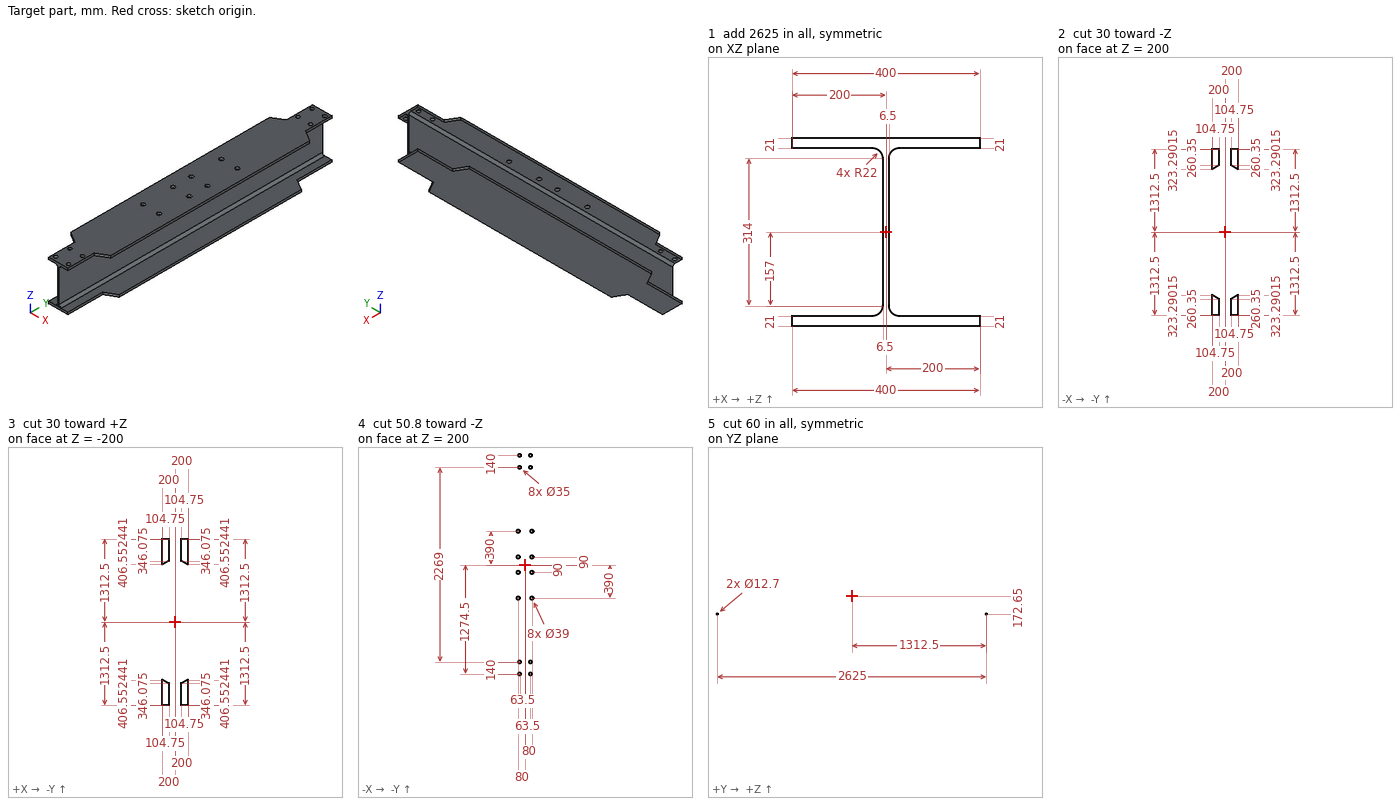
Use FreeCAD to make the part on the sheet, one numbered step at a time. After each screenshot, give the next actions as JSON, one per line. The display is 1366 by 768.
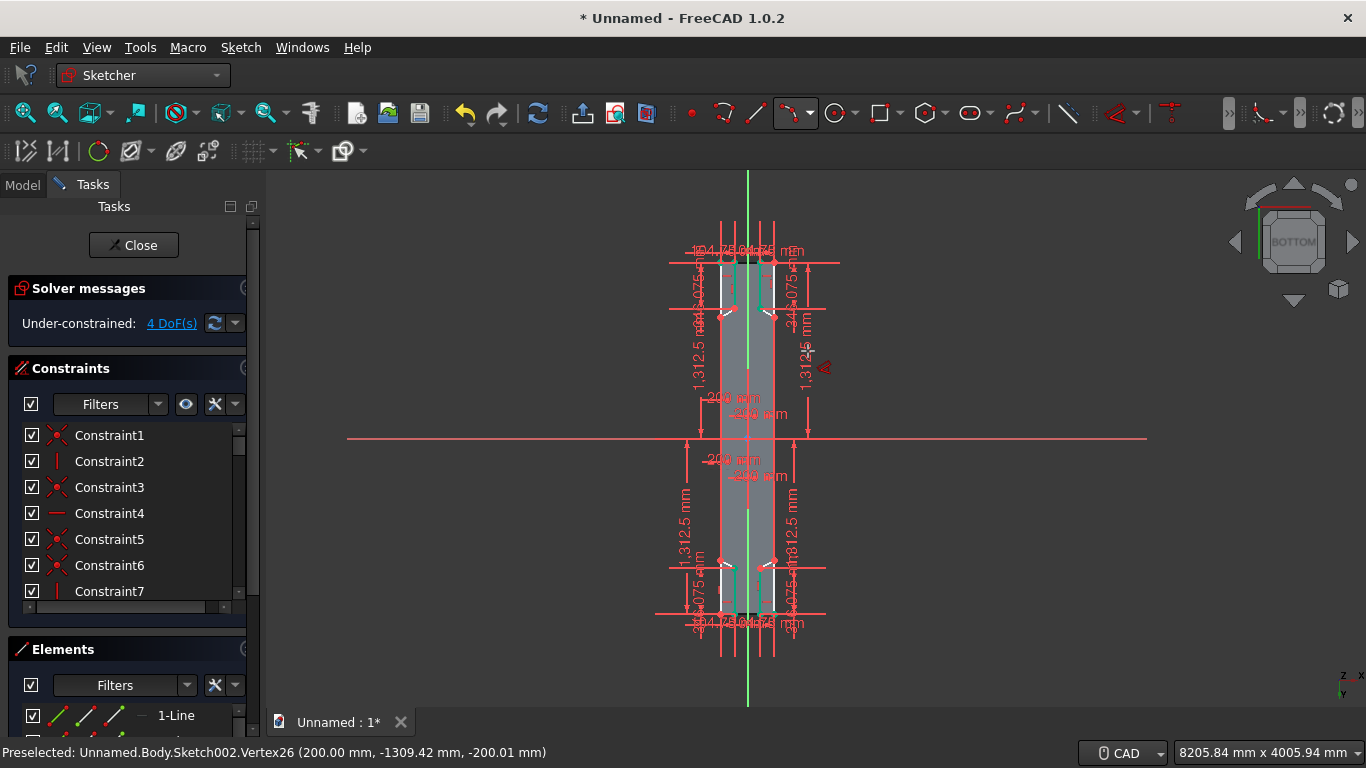
{"action": "left_click", "coordinate": [774, 598]}
{"action": "left_click", "coordinate": [808, 569]}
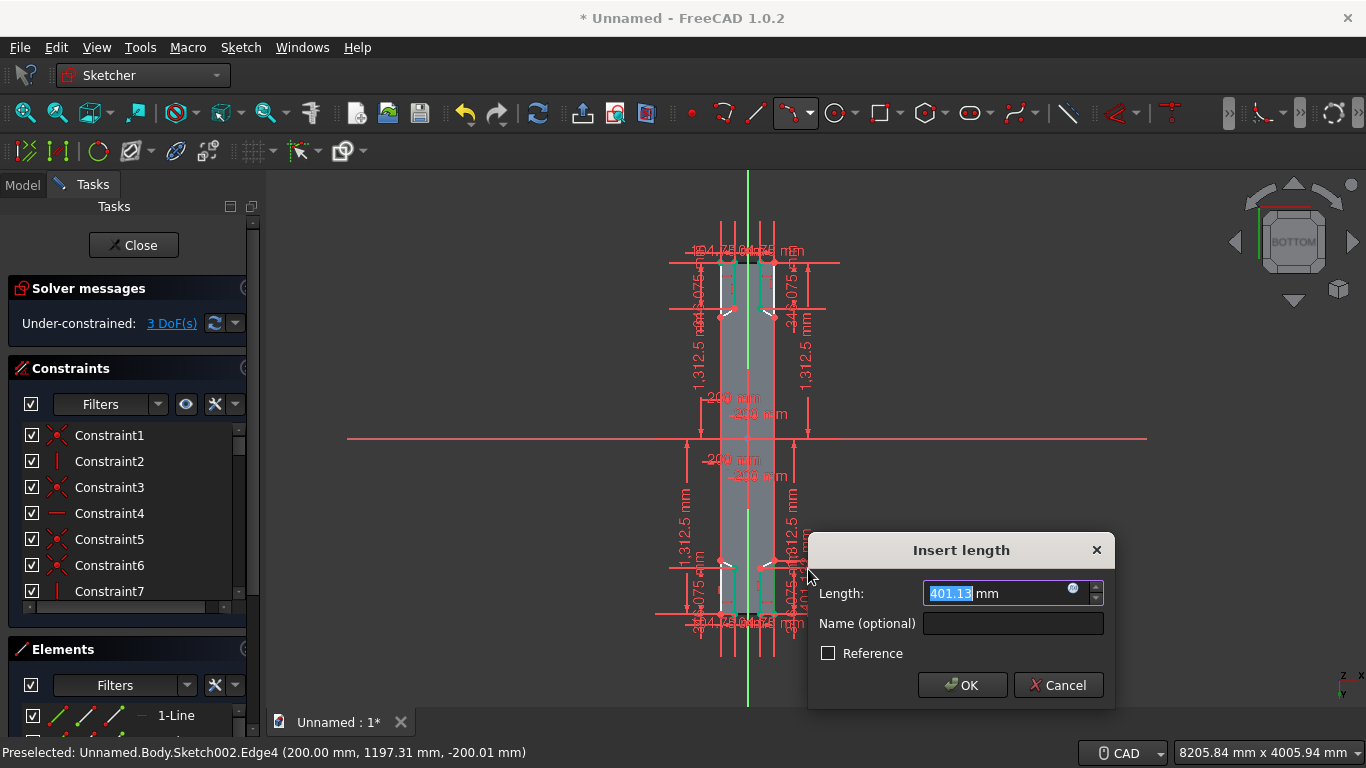
{"action": "type", "text": "406.552441"}
{"action": "key", "text": "Return"}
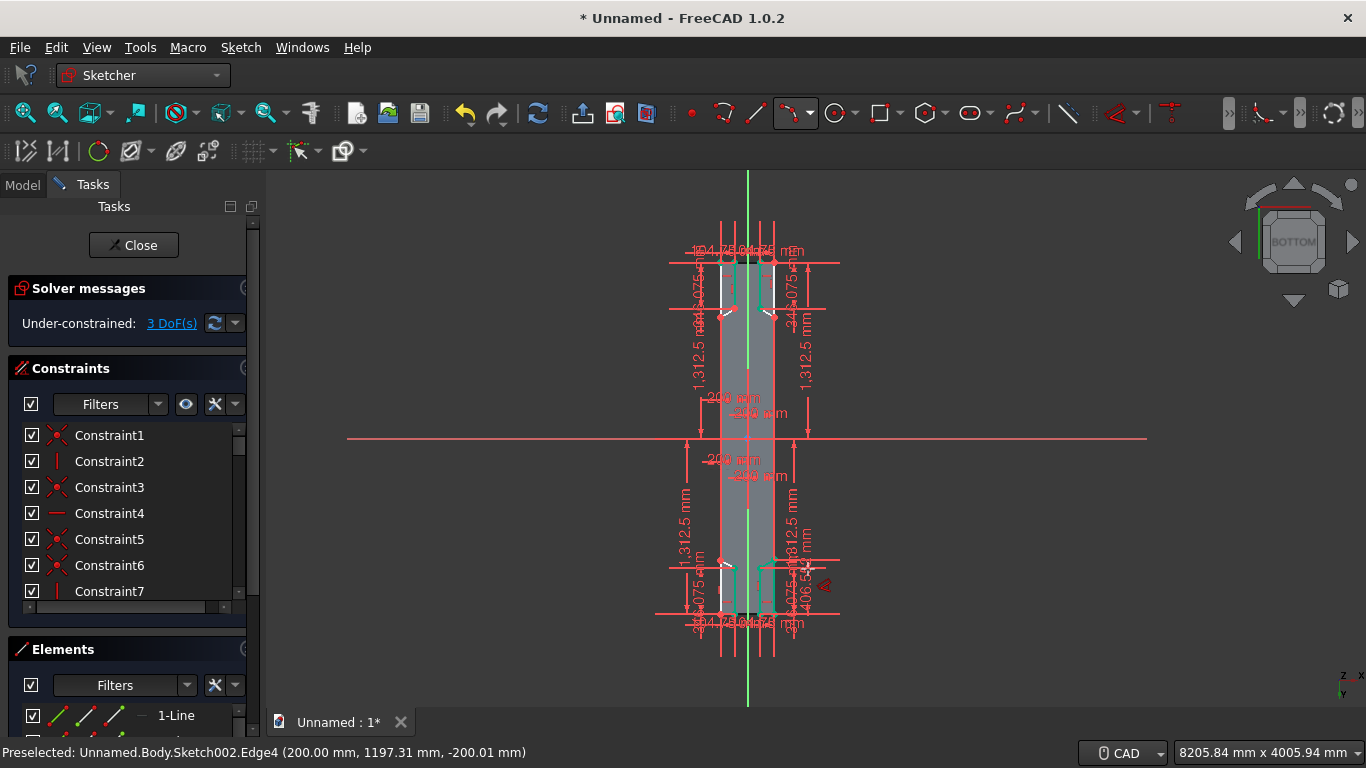
{"action": "left_click", "coordinate": [721, 577]}
{"action": "left_click", "coordinate": [687, 569]}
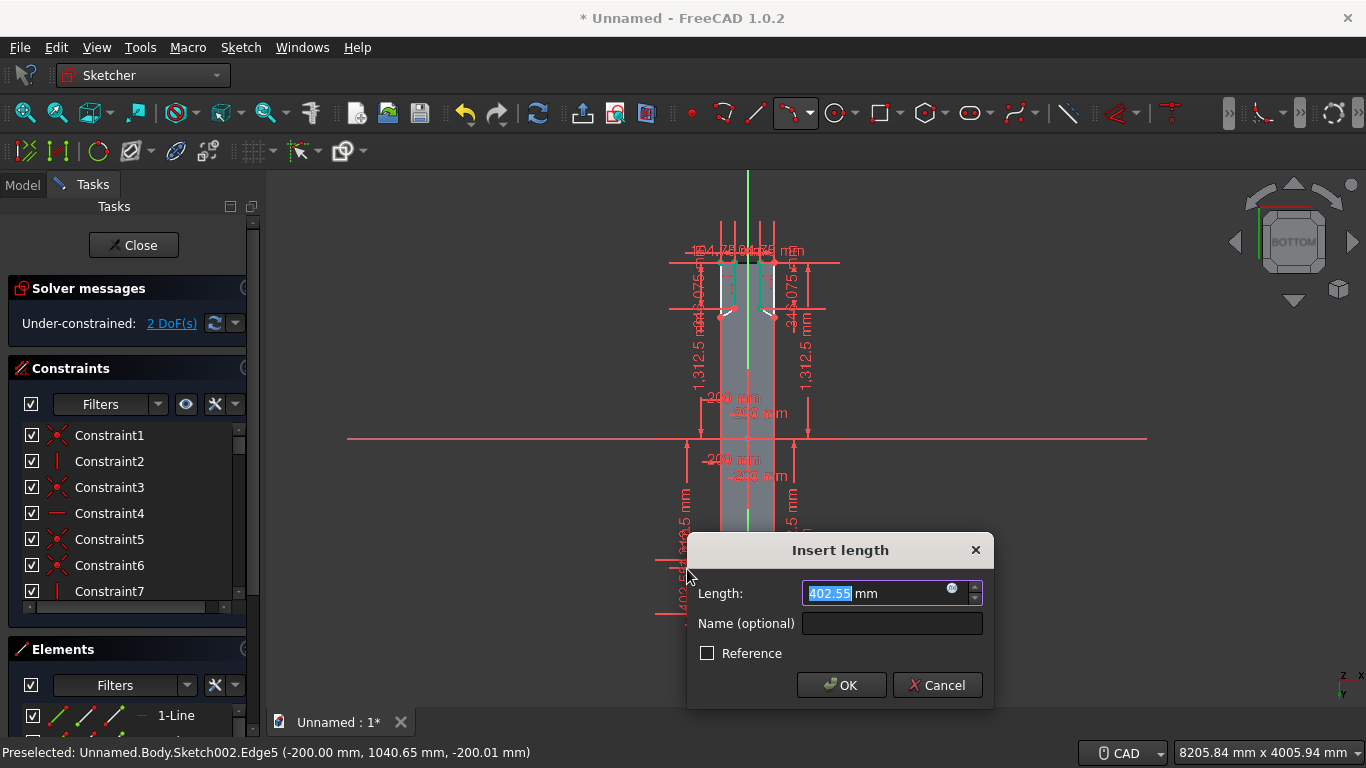
{"action": "type", "text": "406.552441"}
{"action": "key", "text": "Return"}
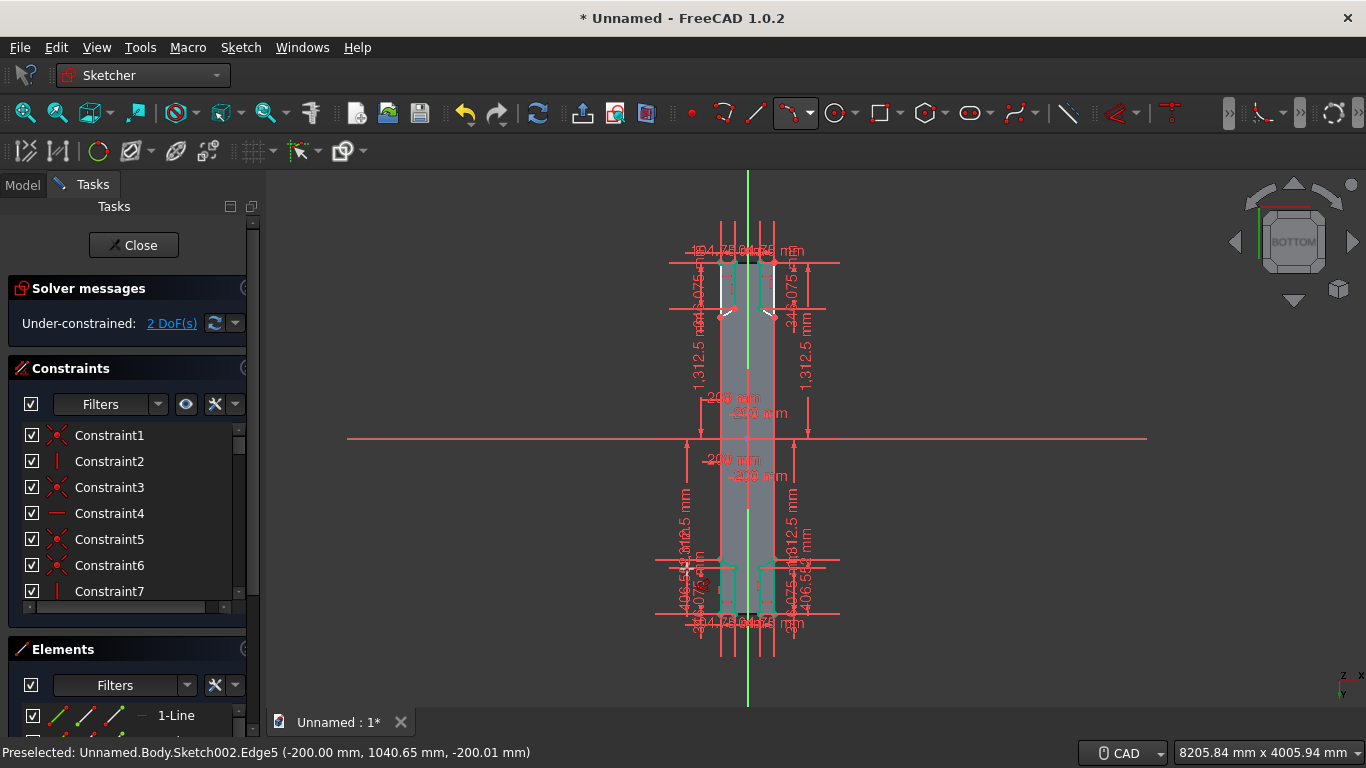
{"action": "left_click", "coordinate": [721, 279]}
{"action": "left_click", "coordinate": [687, 309]}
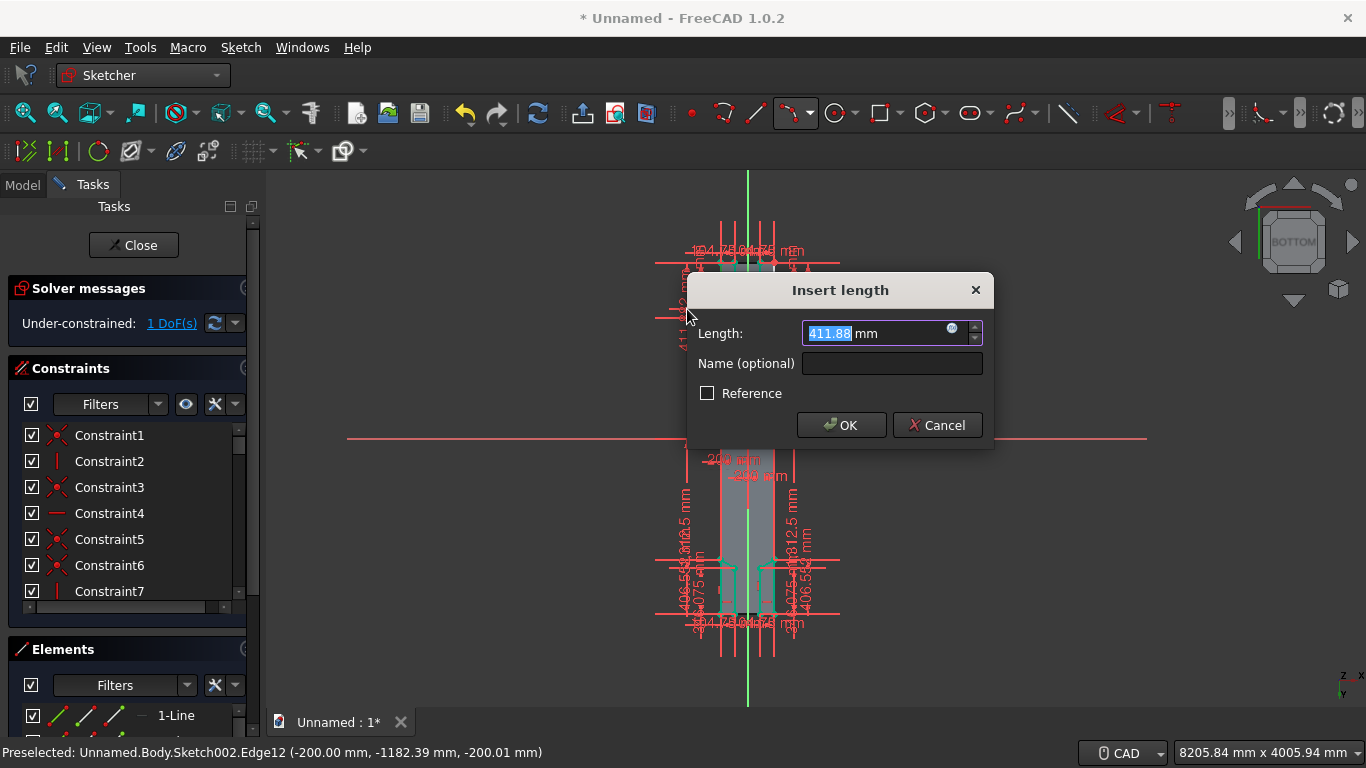
{"action": "type", "text": "406.552441"}
{"action": "key", "text": "Return"}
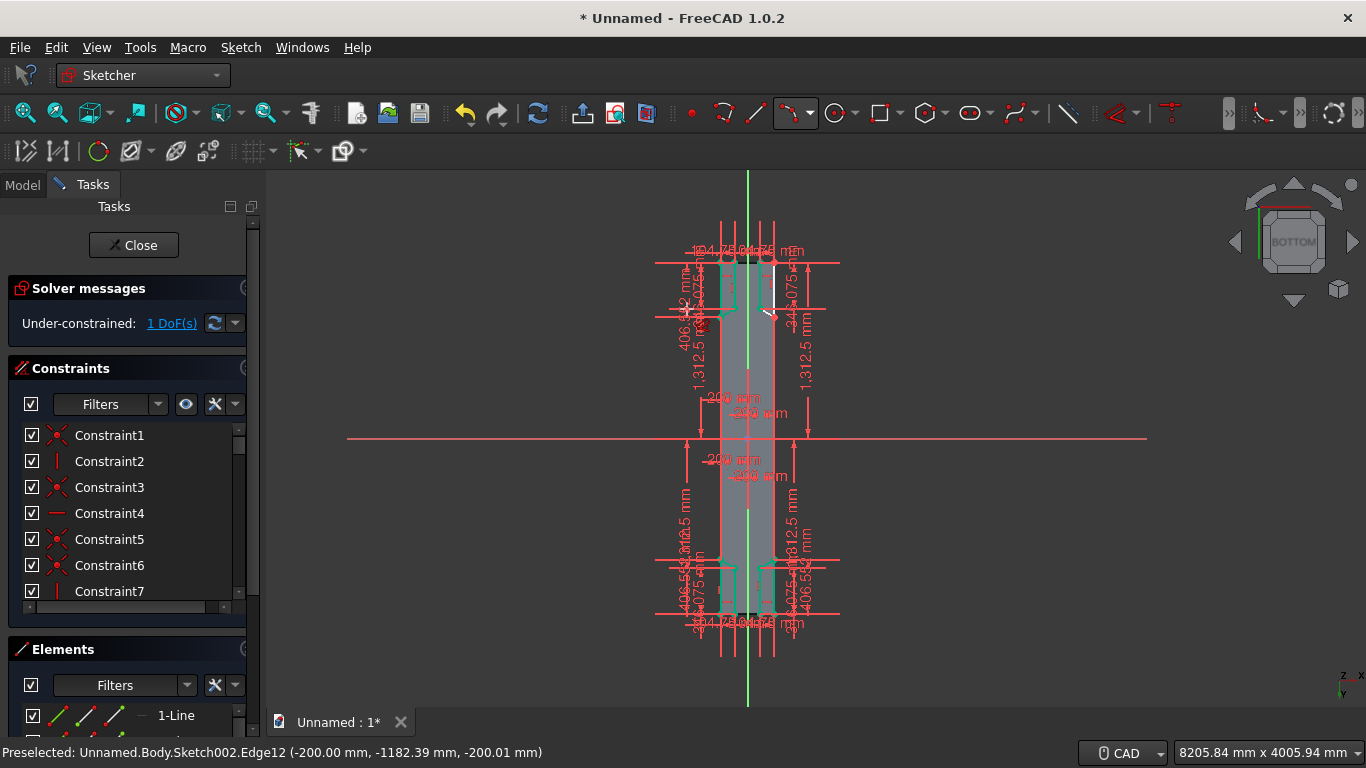
{"action": "left_click", "coordinate": [774, 301]}
{"action": "left_click", "coordinate": [808, 309]}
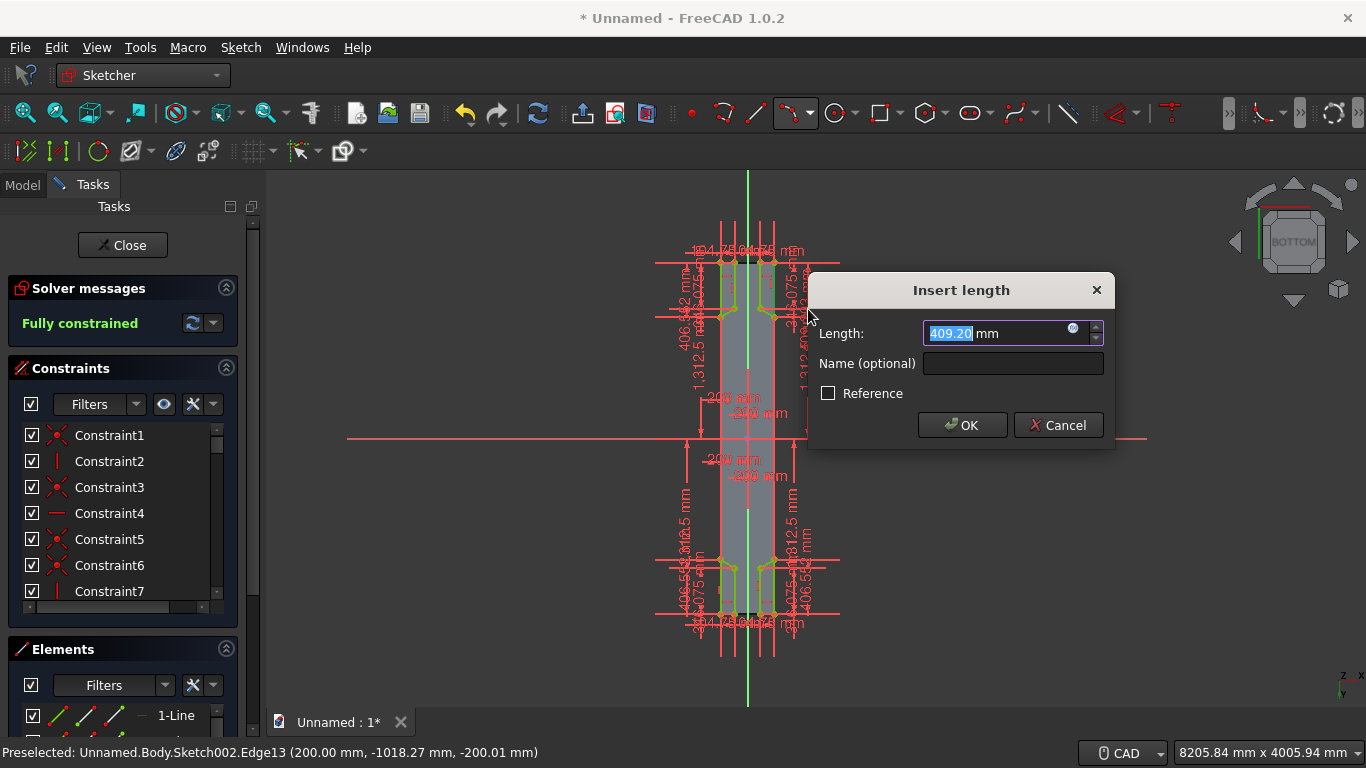
{"action": "type", "text": "406.552441"}
{"action": "key", "text": "Return"}
{"action": "key", "text": "Escape"}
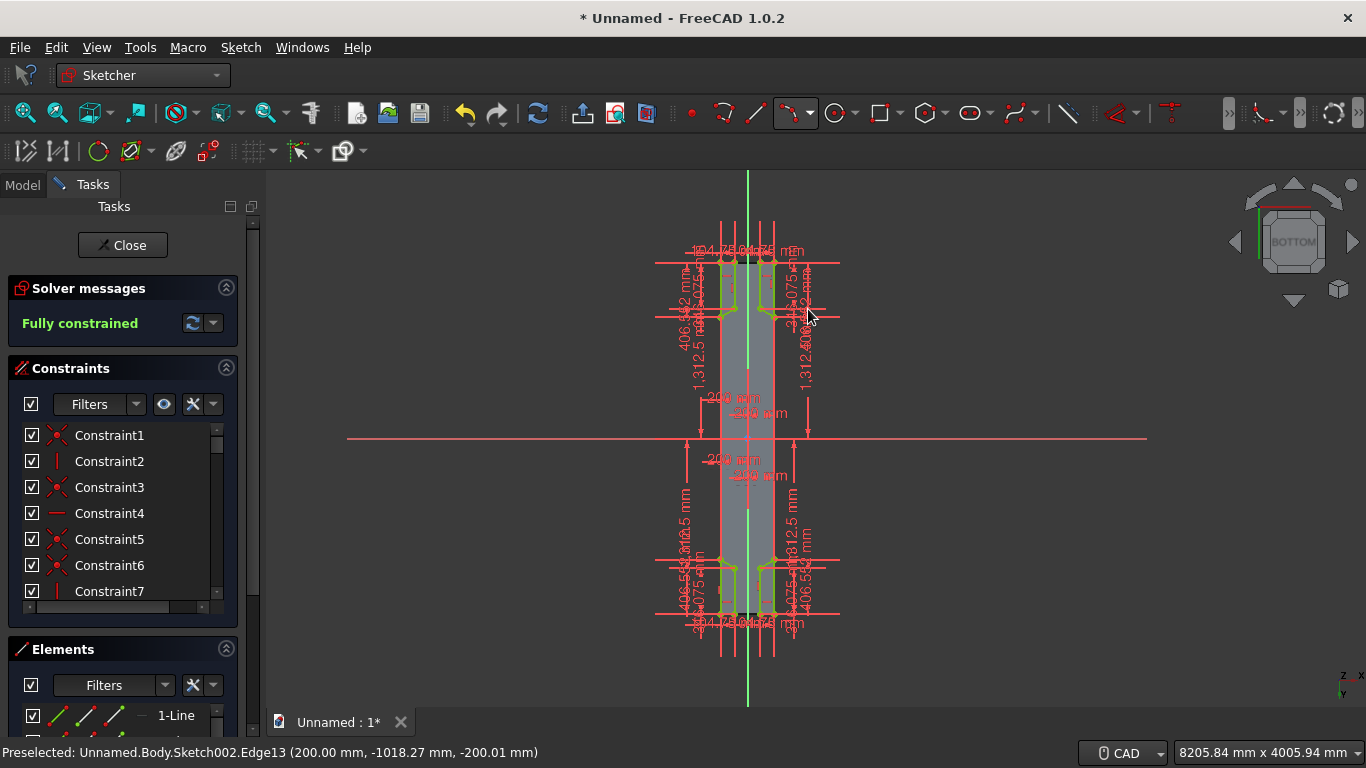
{"action": "left_click", "coordinate": [123, 245]}